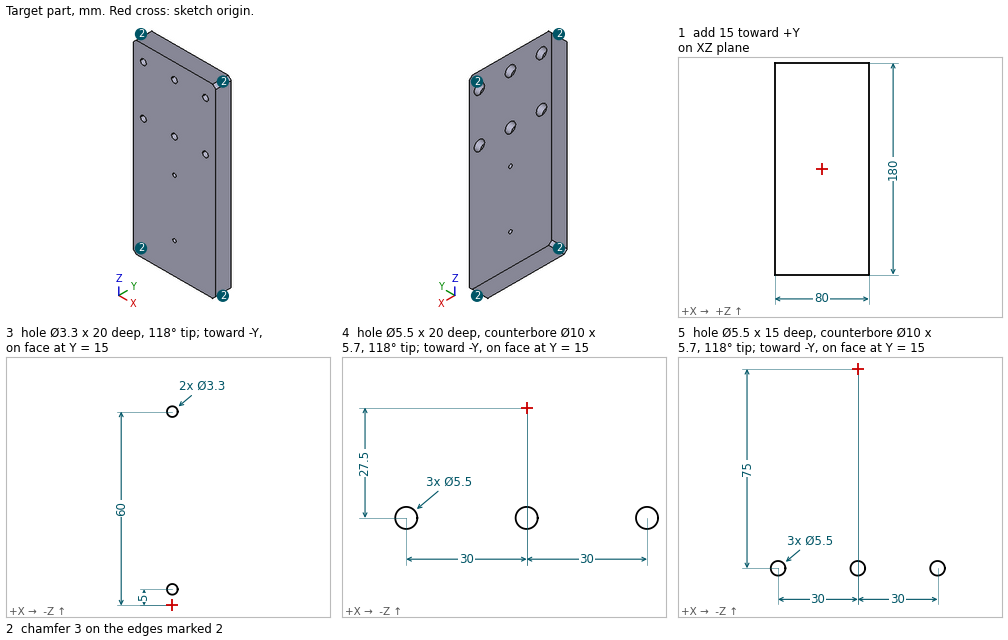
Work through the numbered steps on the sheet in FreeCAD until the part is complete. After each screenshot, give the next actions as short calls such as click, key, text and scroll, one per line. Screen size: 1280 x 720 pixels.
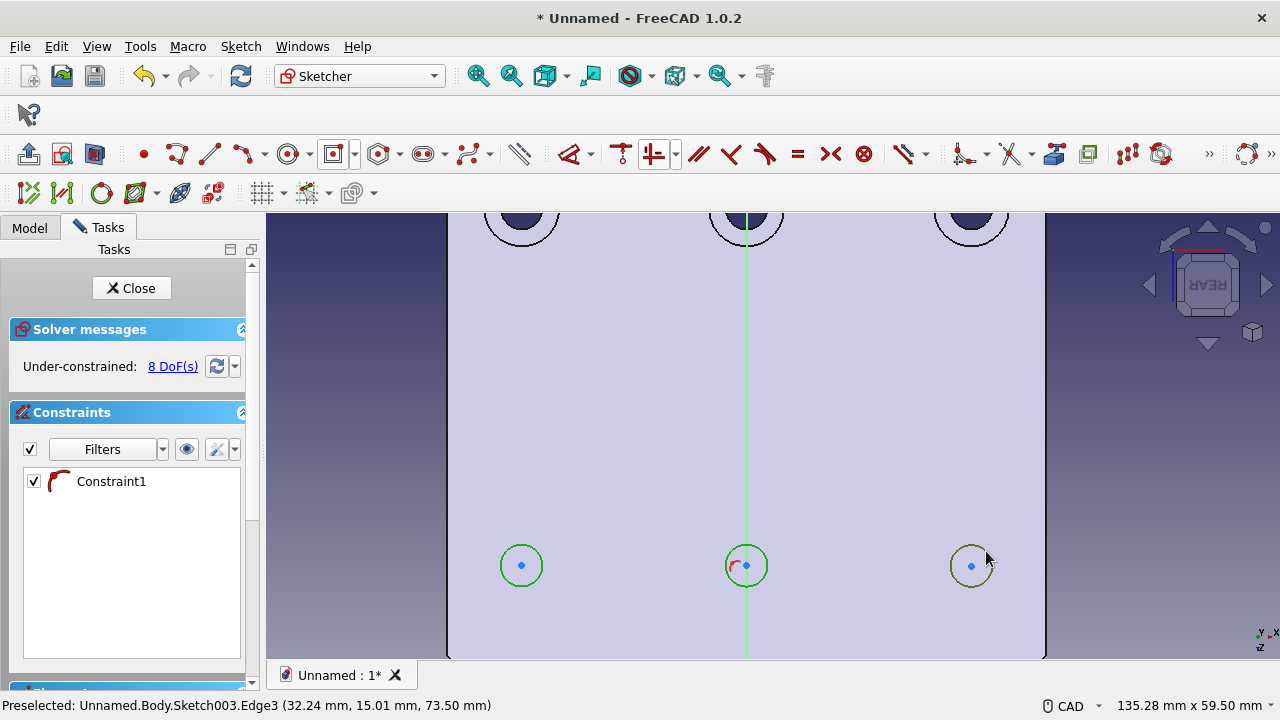
click(798, 154)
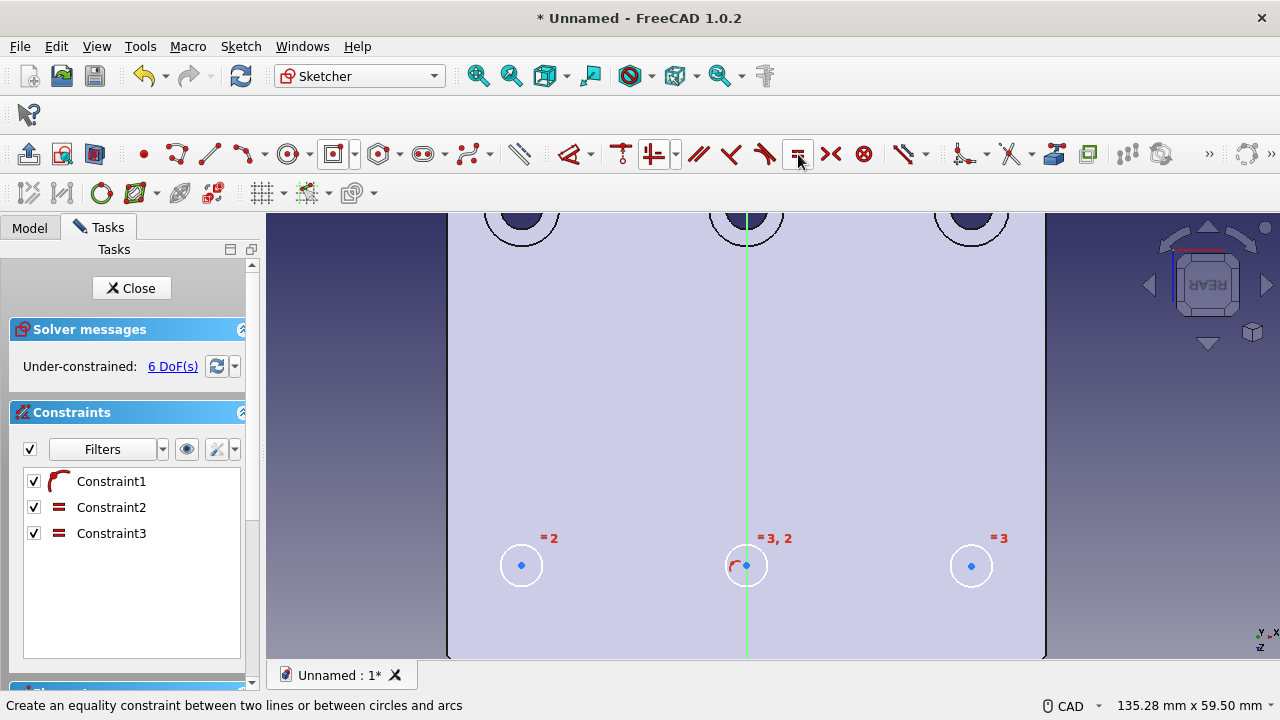
click(522, 566)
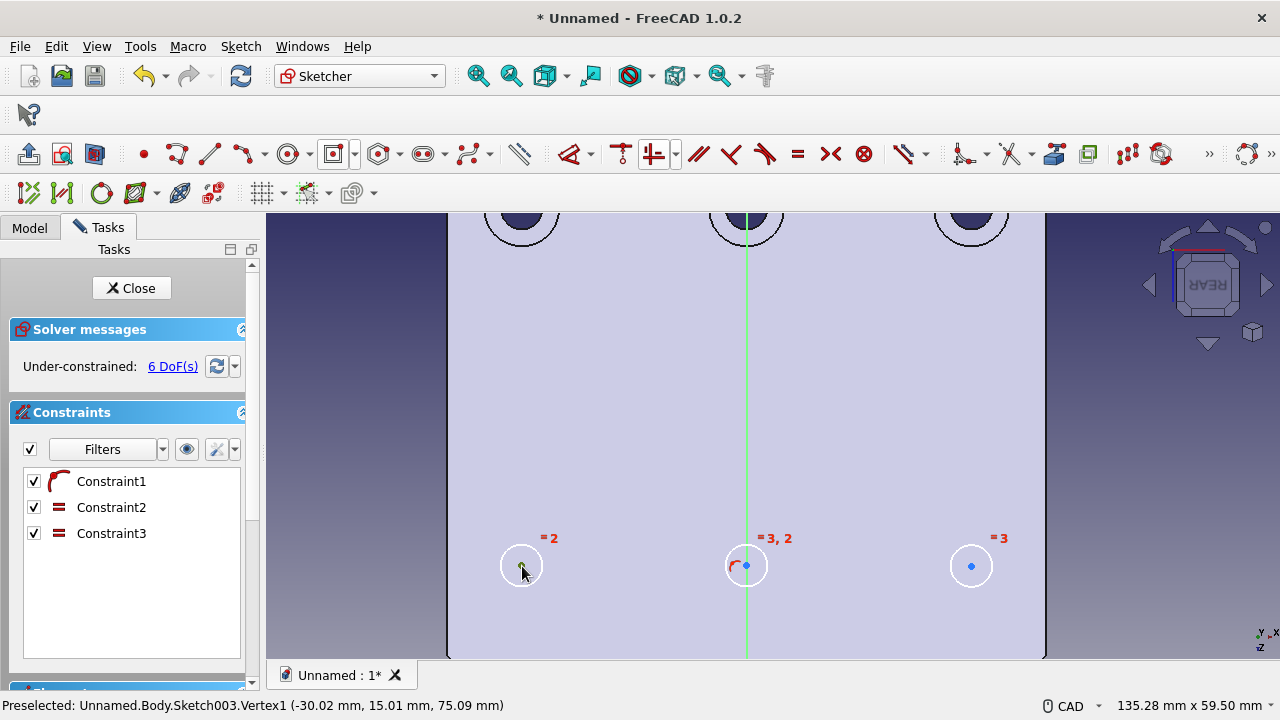
click(747, 566)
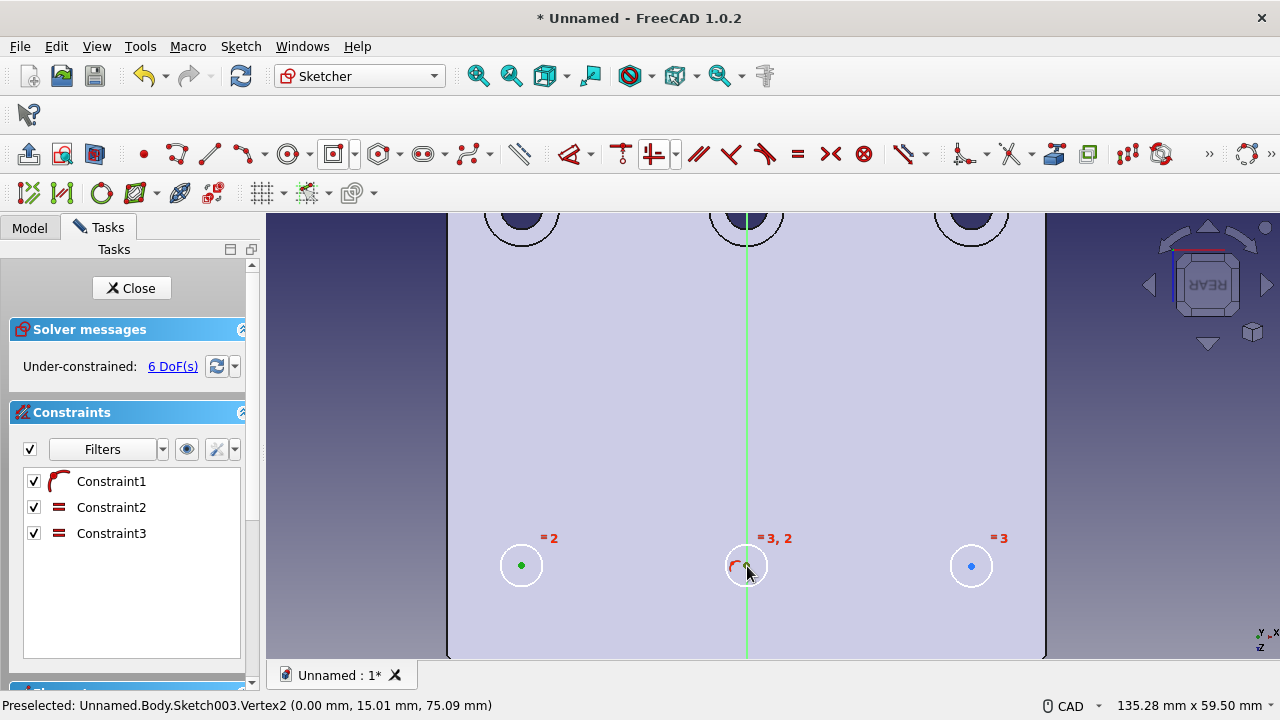
key(h)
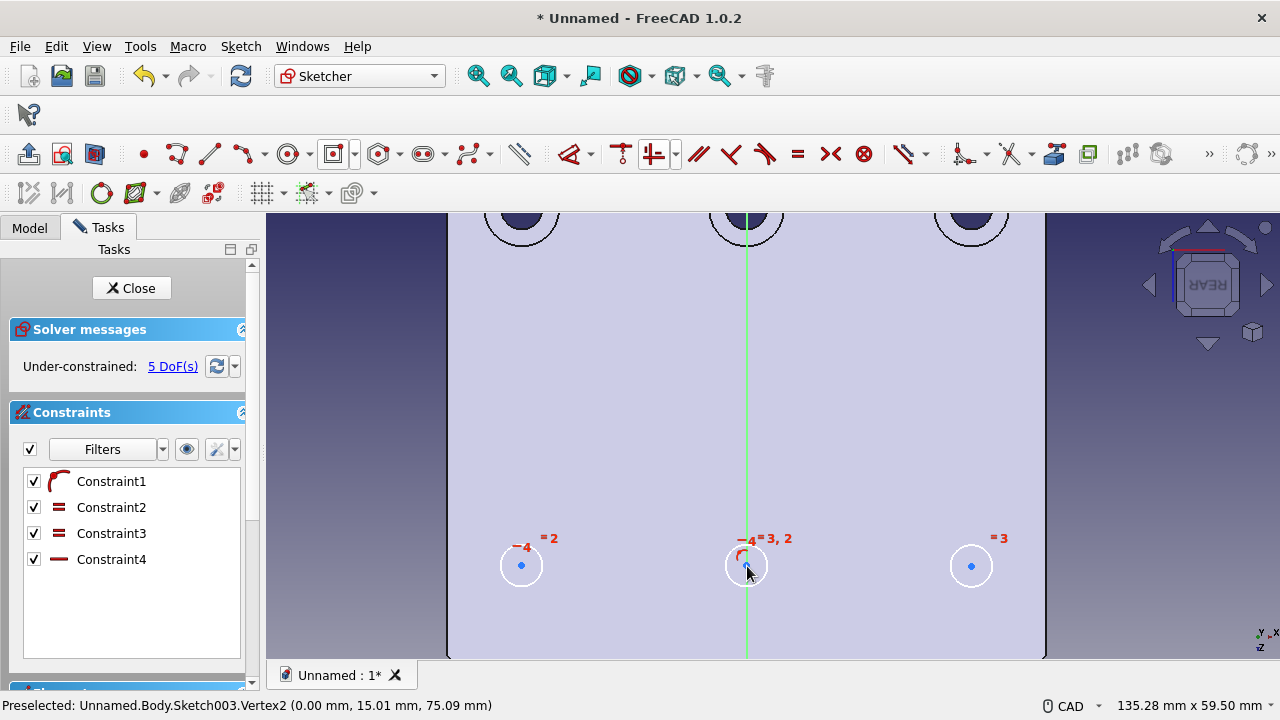
click(747, 566)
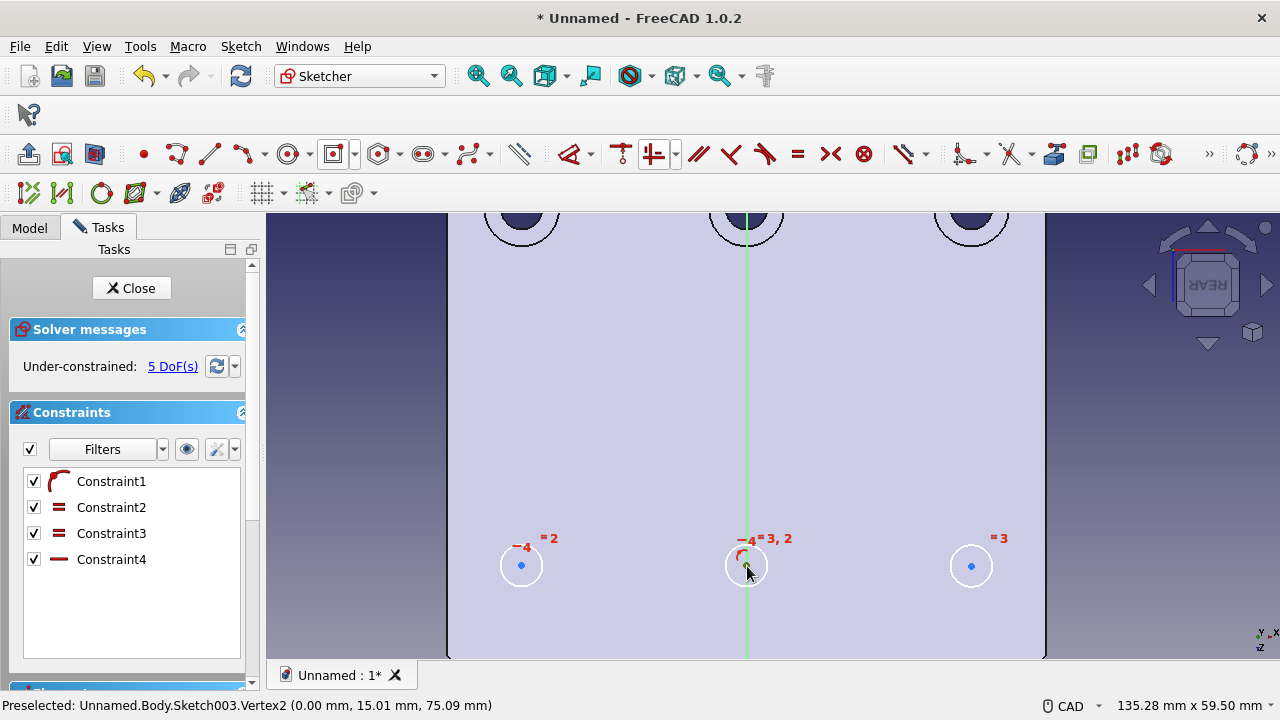
click(971, 566)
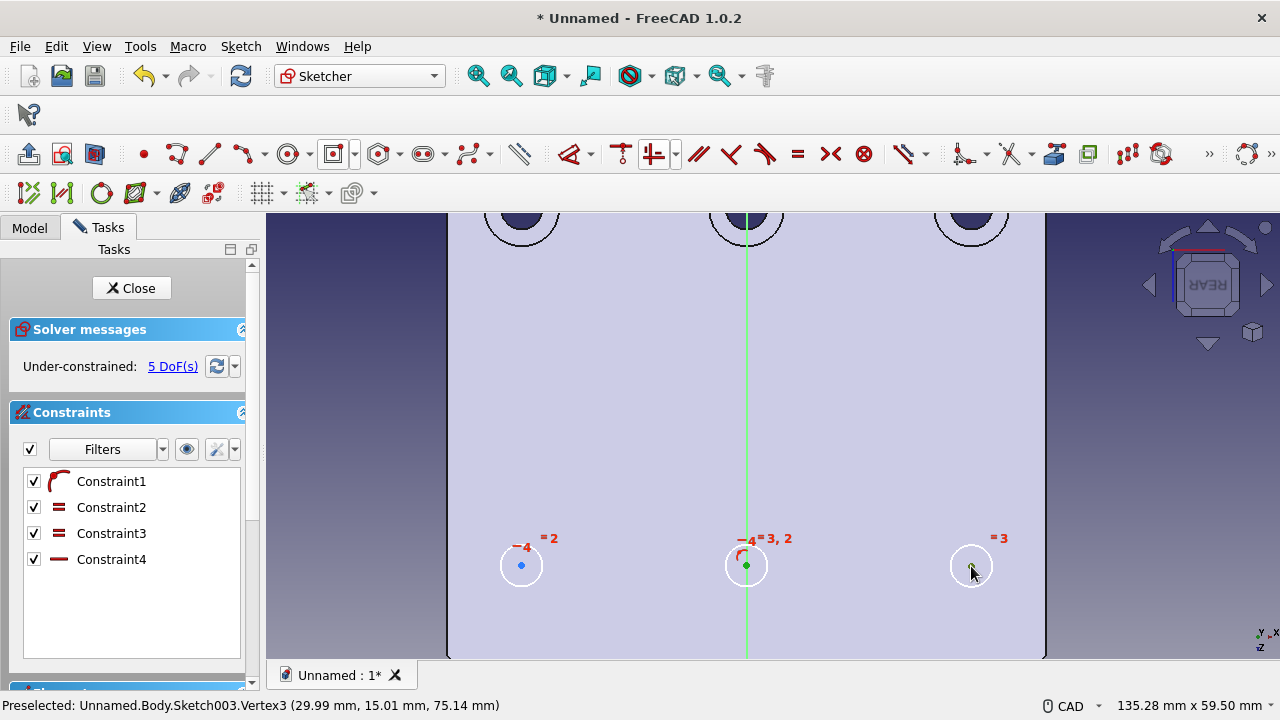
click(676, 154)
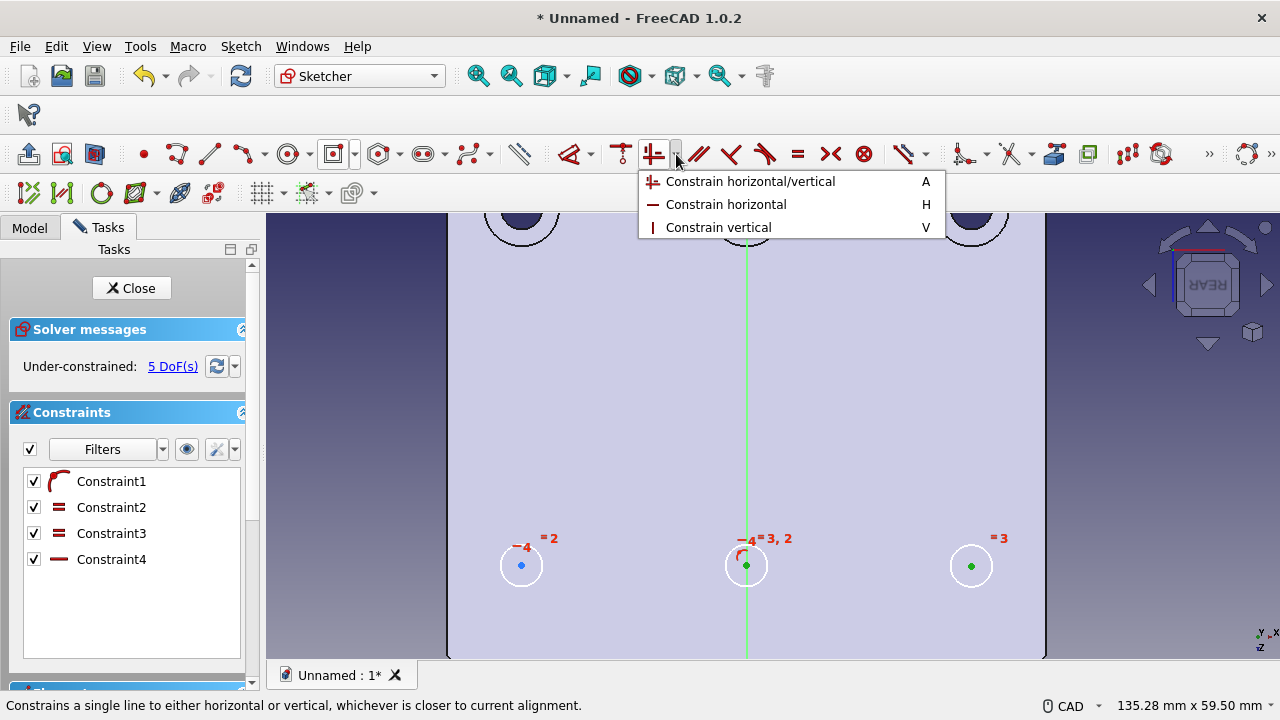
click(792, 204)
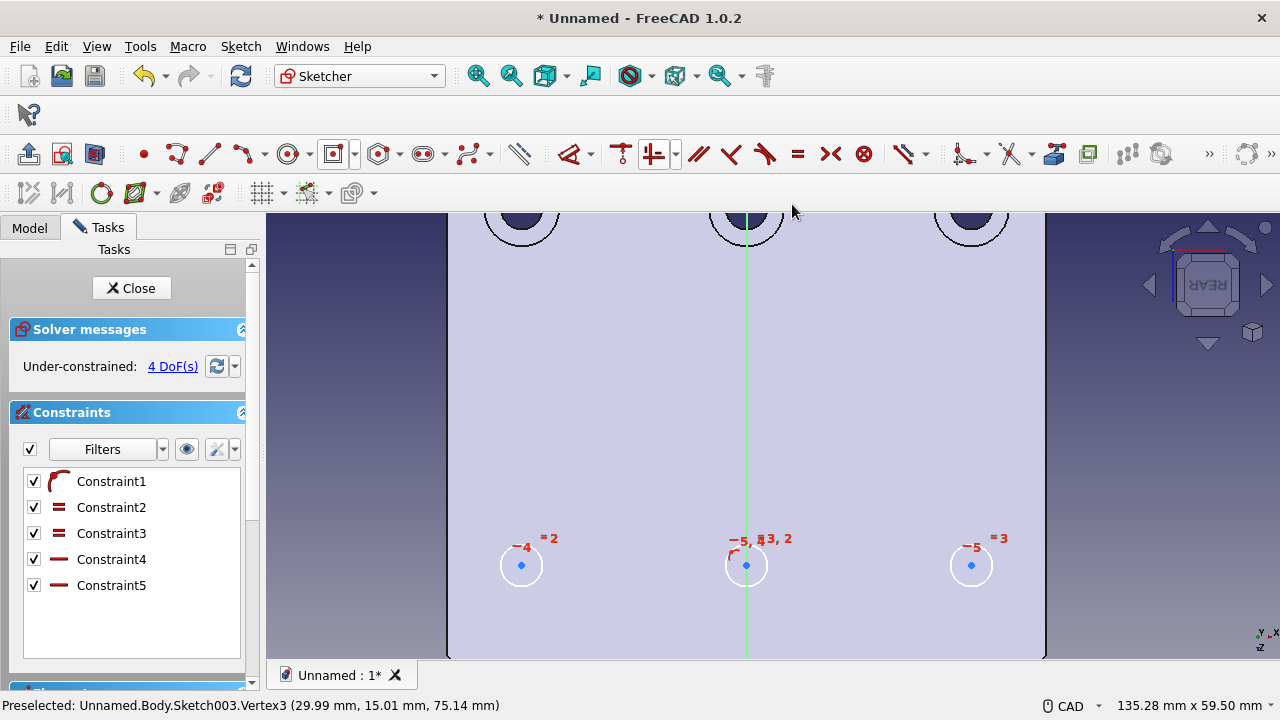
click(568, 154)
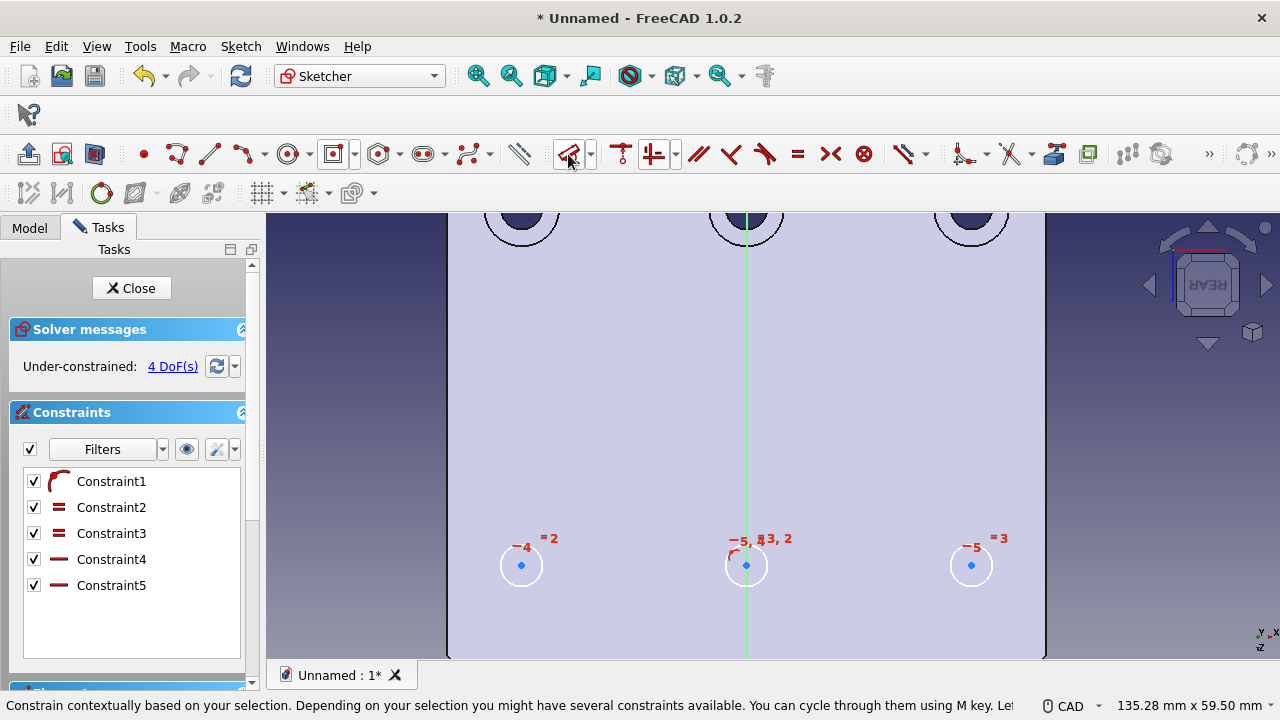
click(536, 551)
click(558, 528)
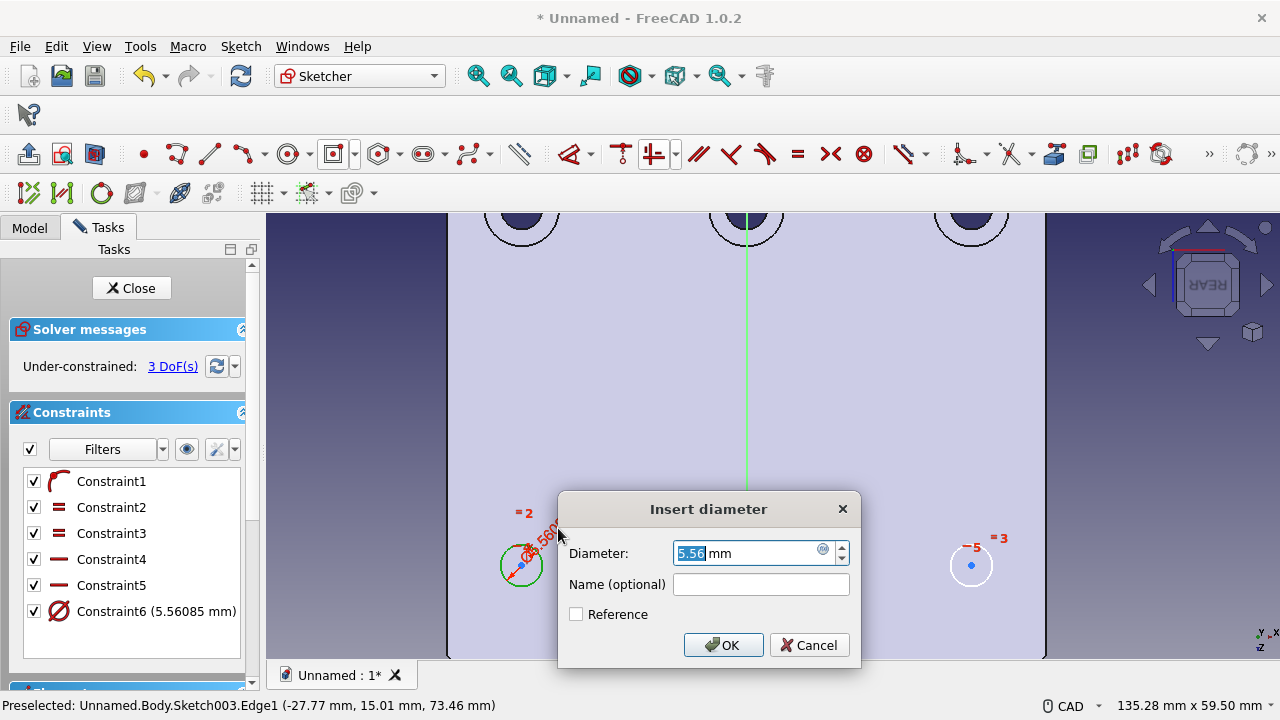
text(5.5)
key(Return)